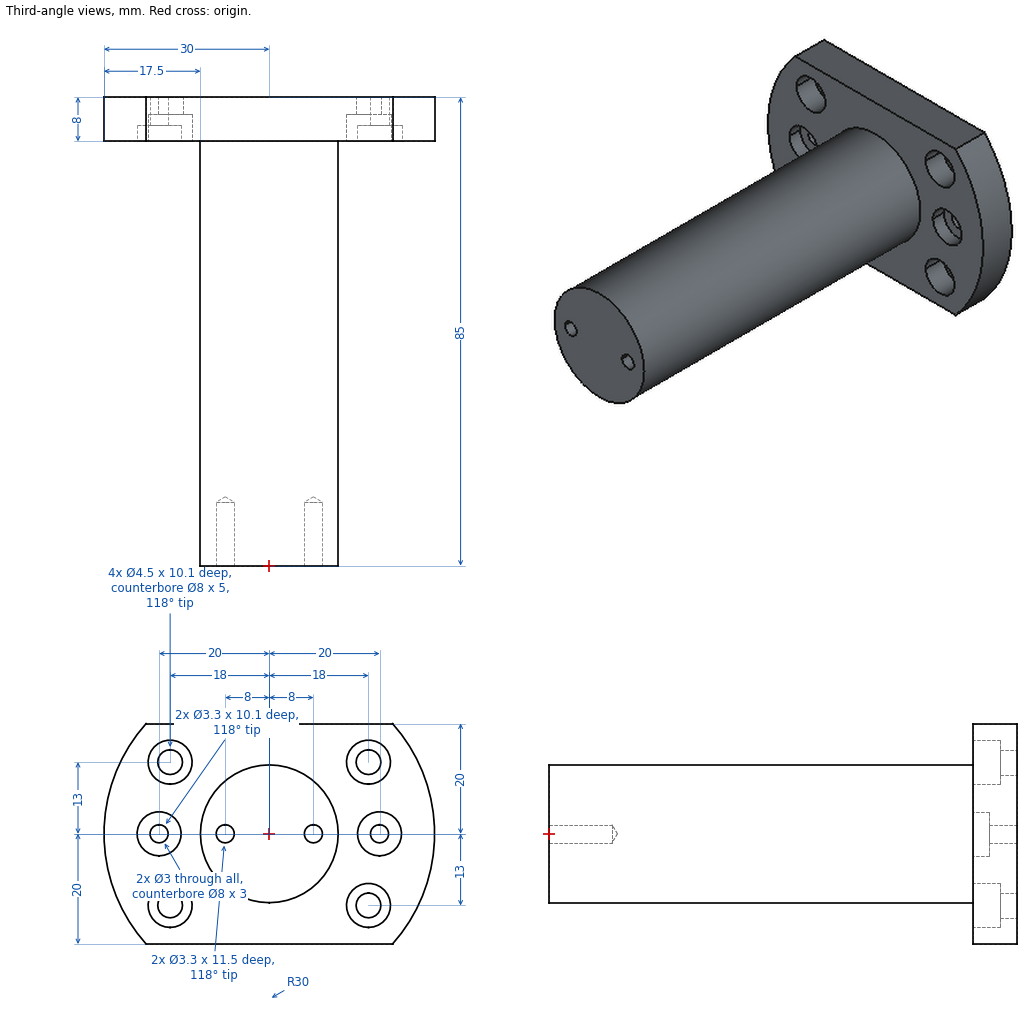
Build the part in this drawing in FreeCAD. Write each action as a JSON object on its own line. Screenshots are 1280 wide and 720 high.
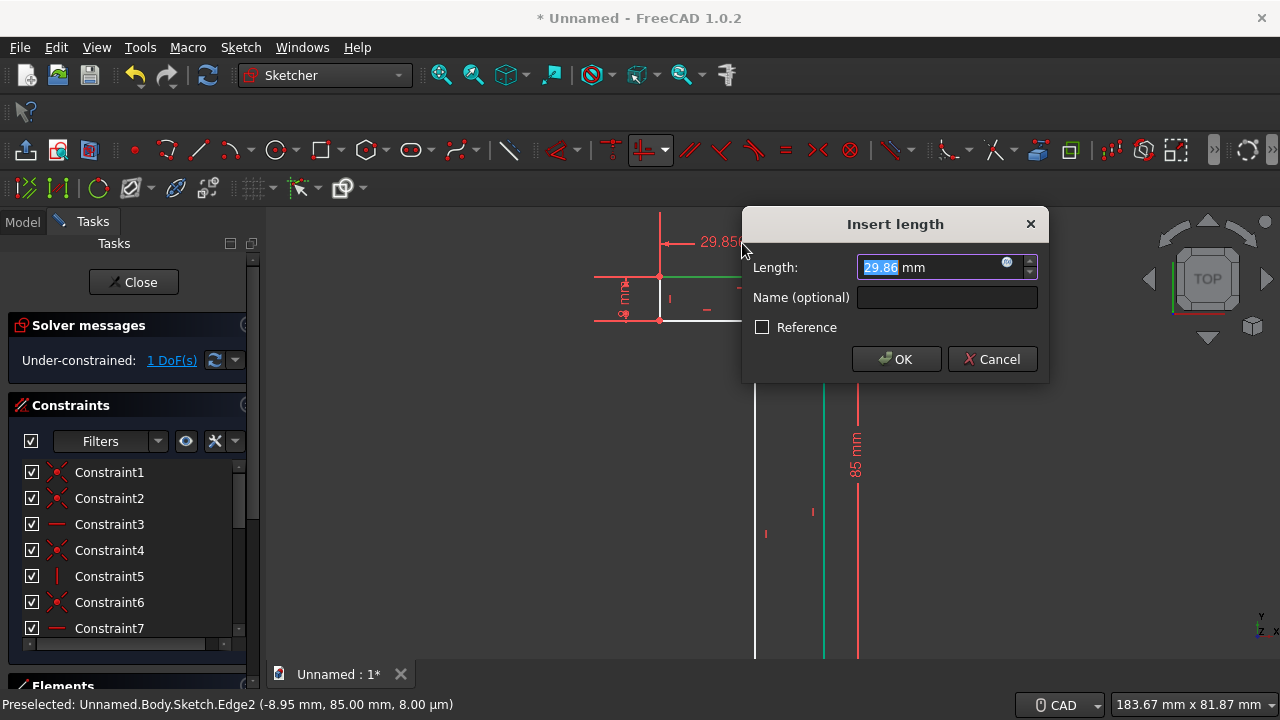
{"action": "type", "text": "30"}
{"action": "key", "text": "Return"}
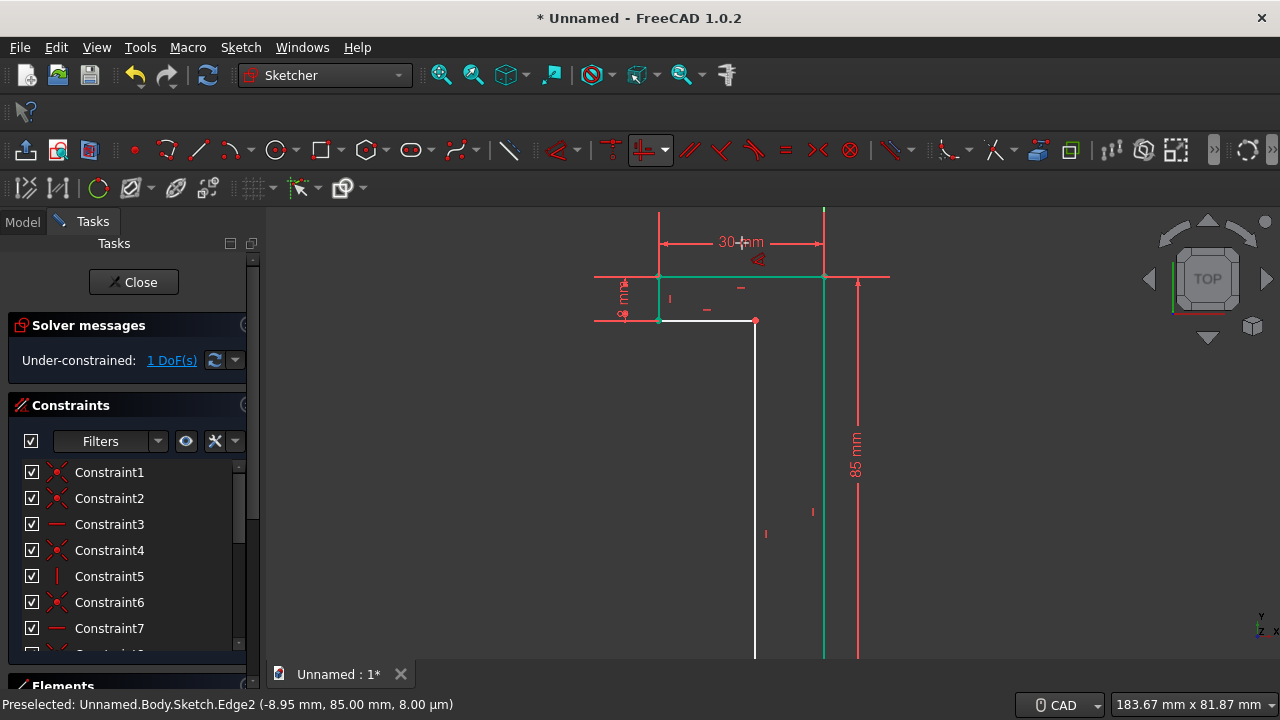
{"action": "left_click", "coordinate": [688, 321]}
{"action": "left_click", "coordinate": [707, 355]}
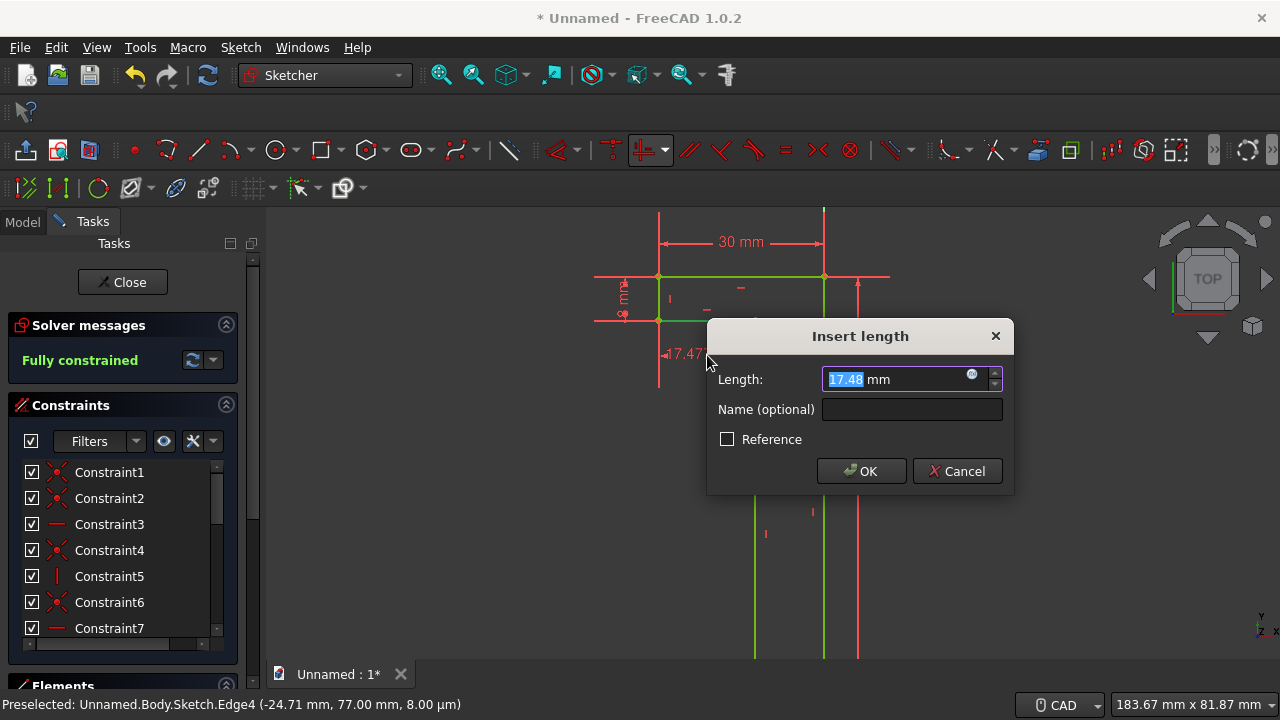
{"action": "type", "text": "17.5"}
{"action": "key", "text": "Return"}
{"action": "key", "text": "Escape"}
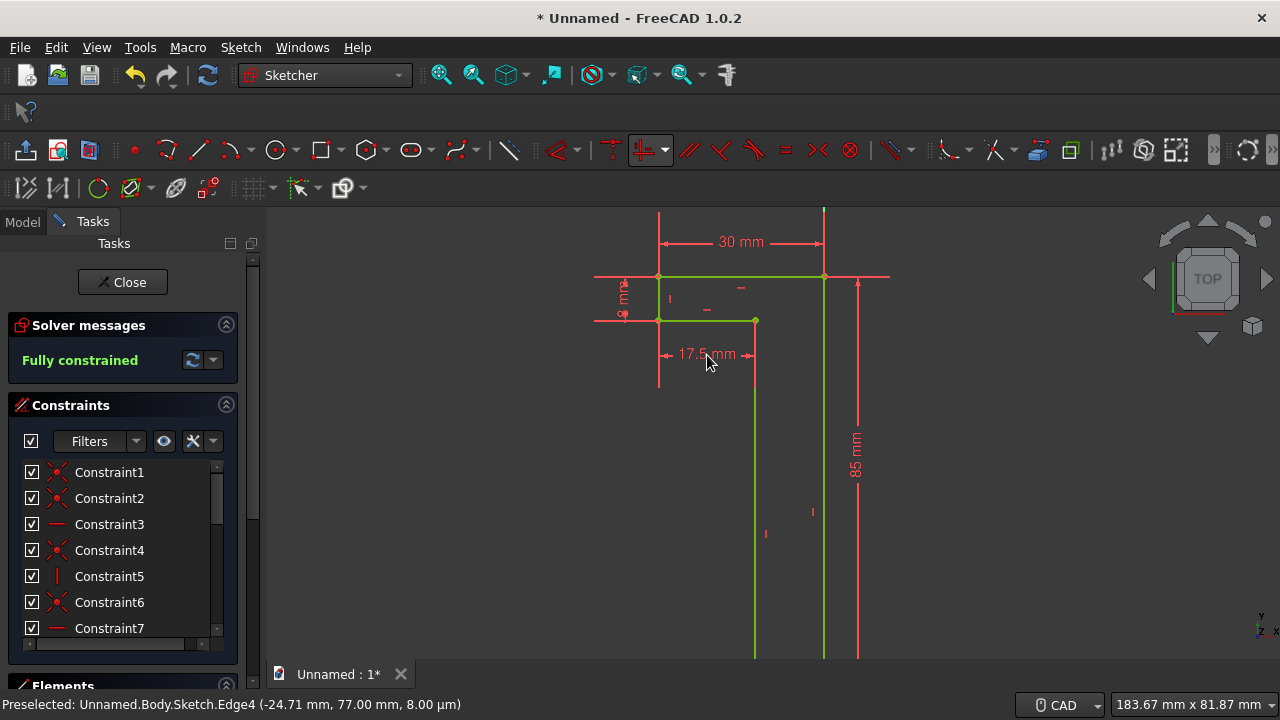
{"action": "left_click", "coordinate": [123, 282]}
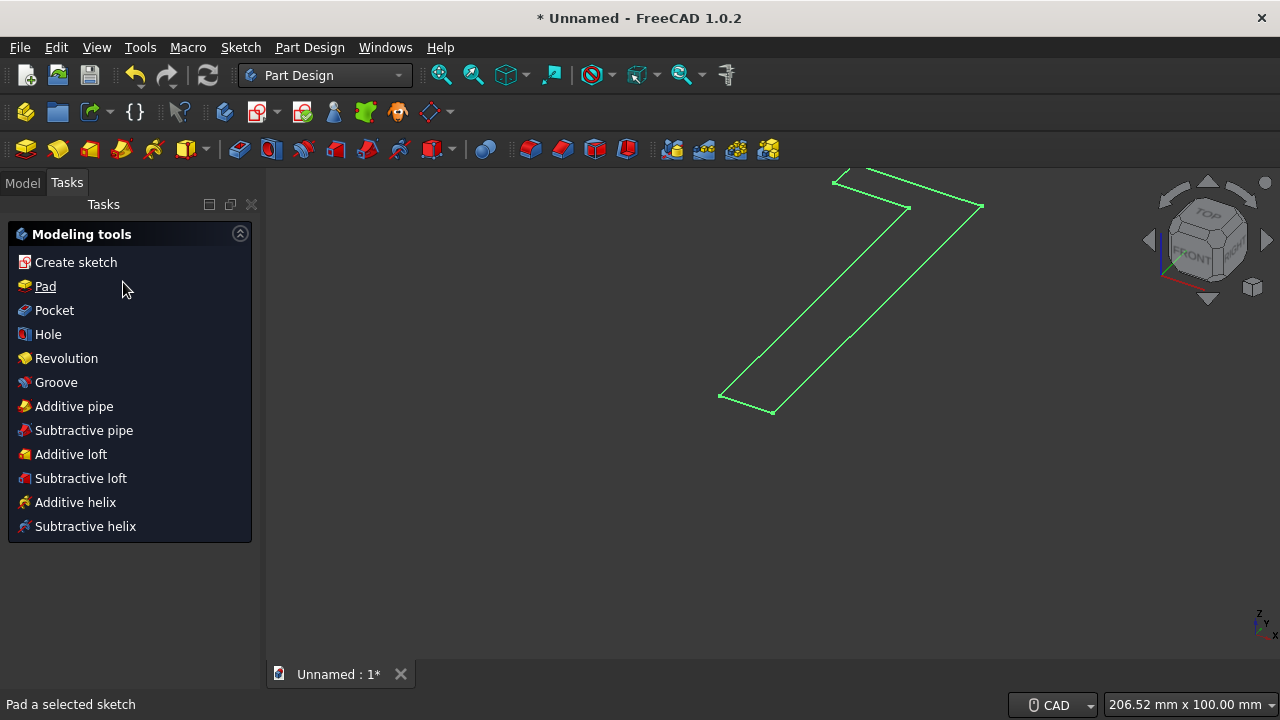
{"action": "left_click", "coordinate": [58, 150]}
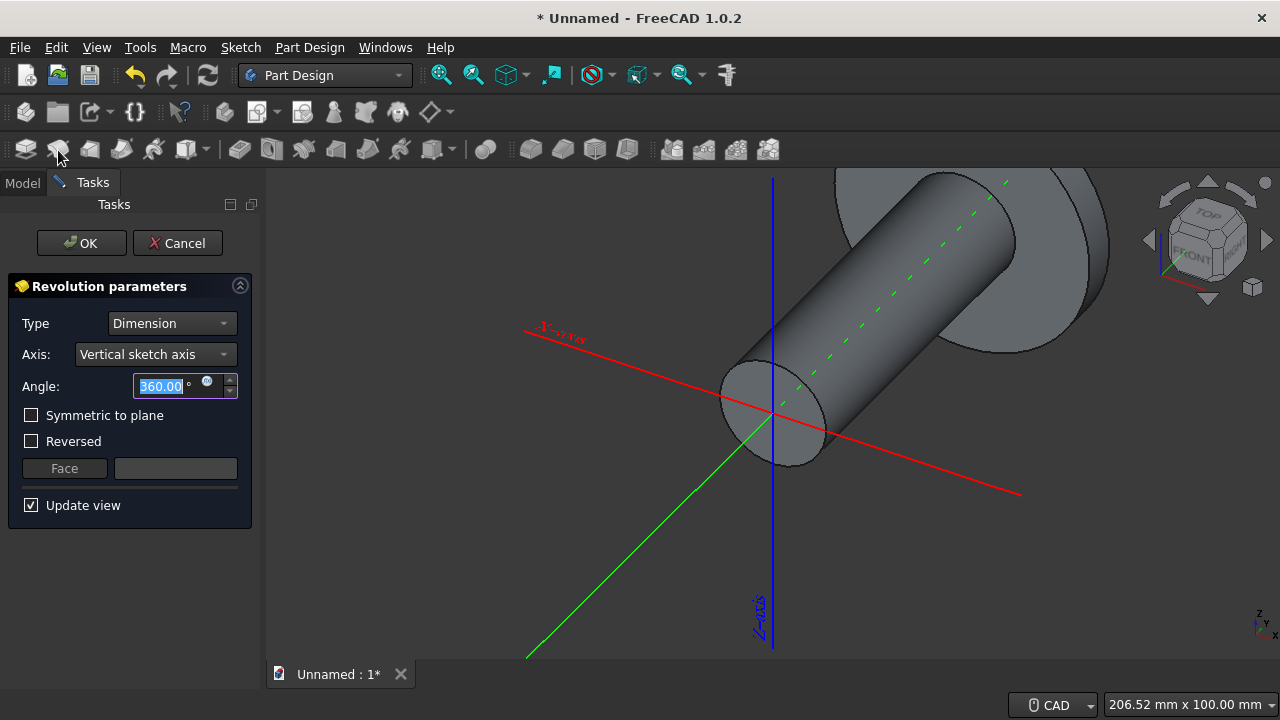
{"action": "left_click", "coordinate": [82, 243]}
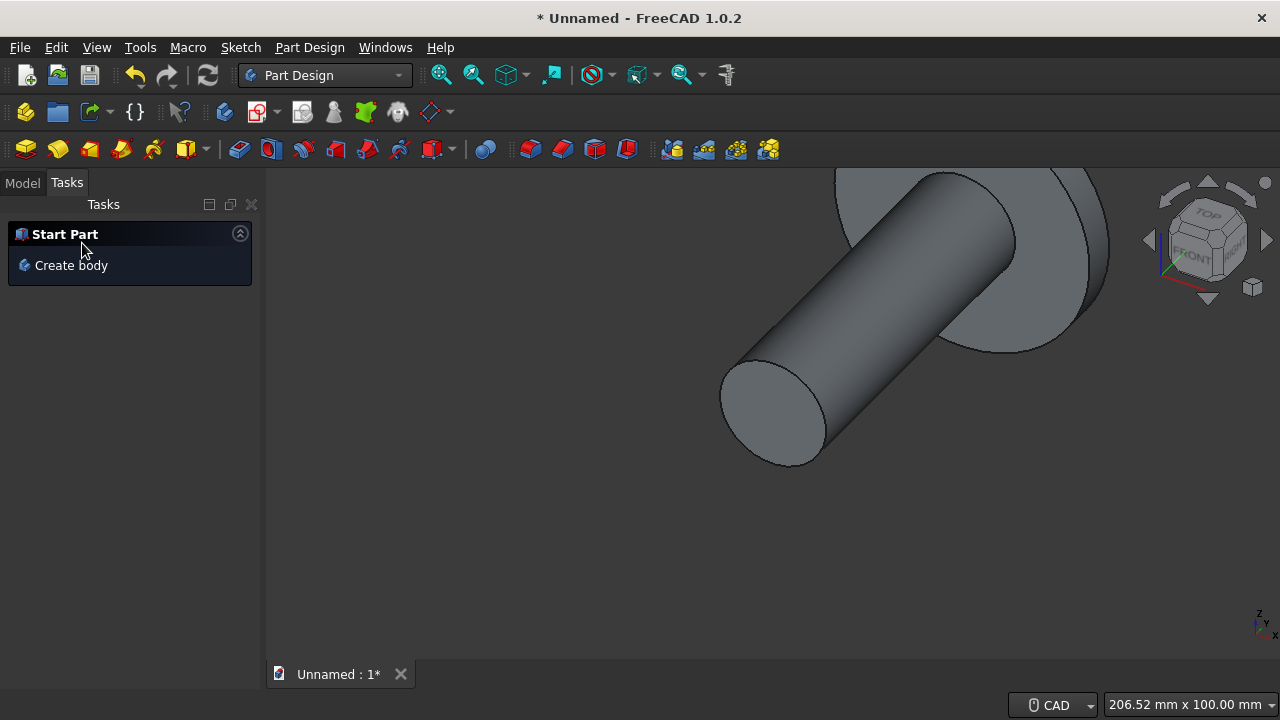
{"action": "left_click", "coordinate": [442, 76]}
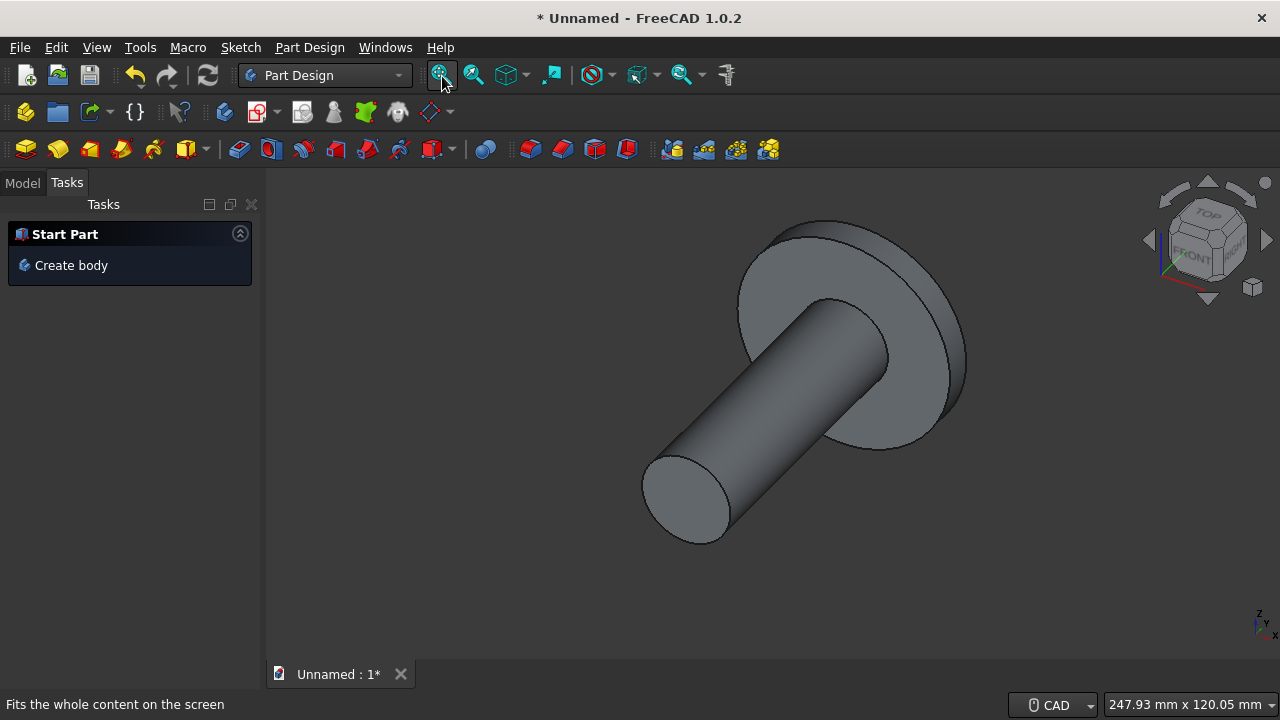
{"action": "left_click", "coordinate": [686, 499]}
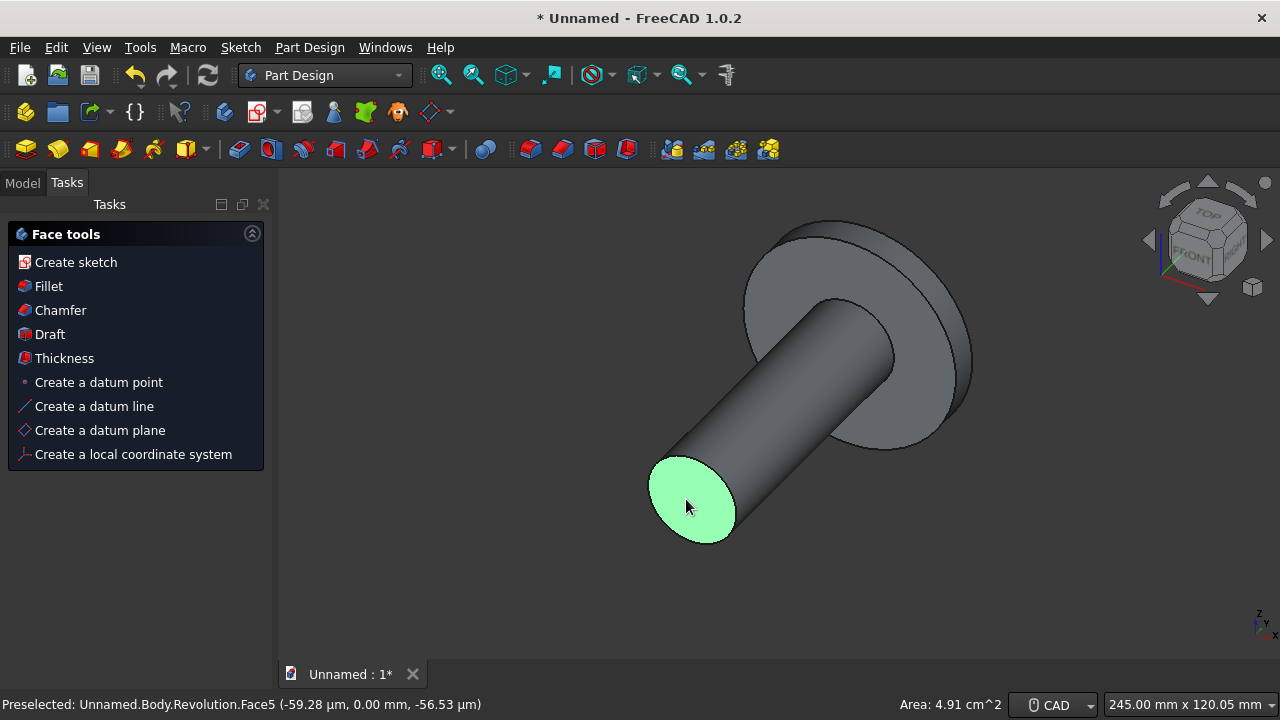
{"action": "left_click", "coordinate": [258, 112]}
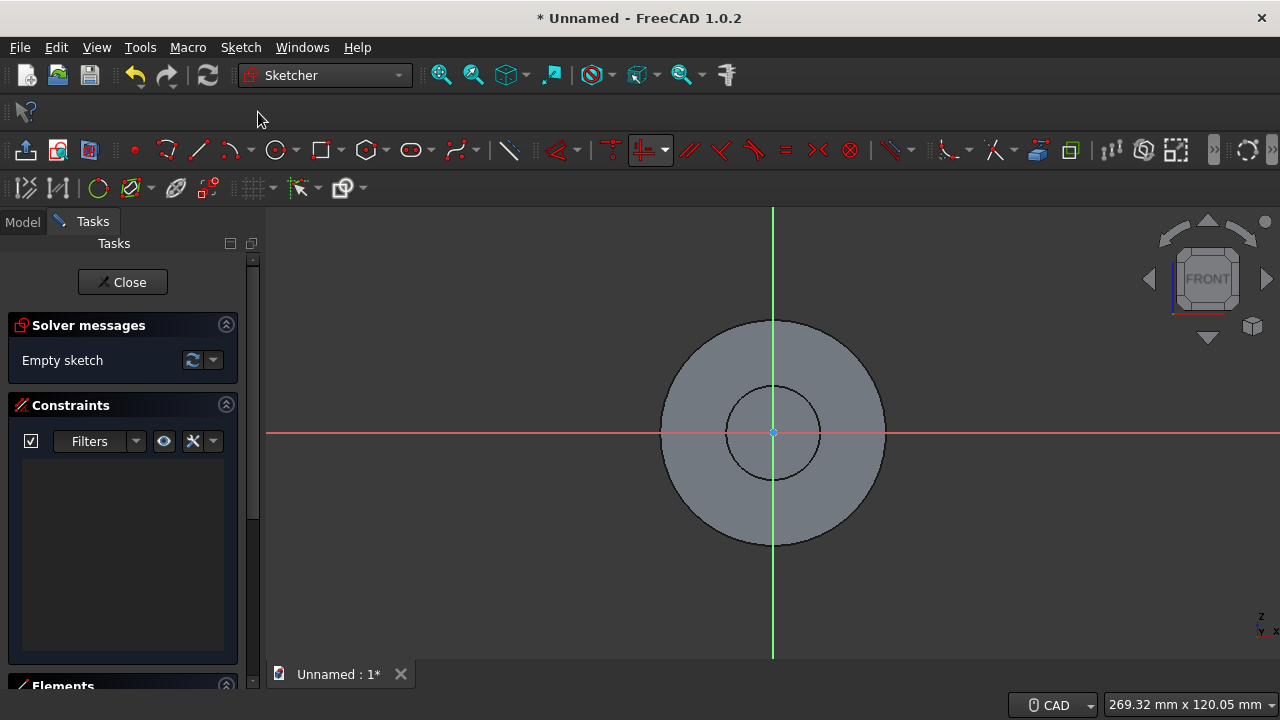
{"action": "scroll", "coordinate": [784, 433], "scroll_direction": "up", "scroll_amount": 10}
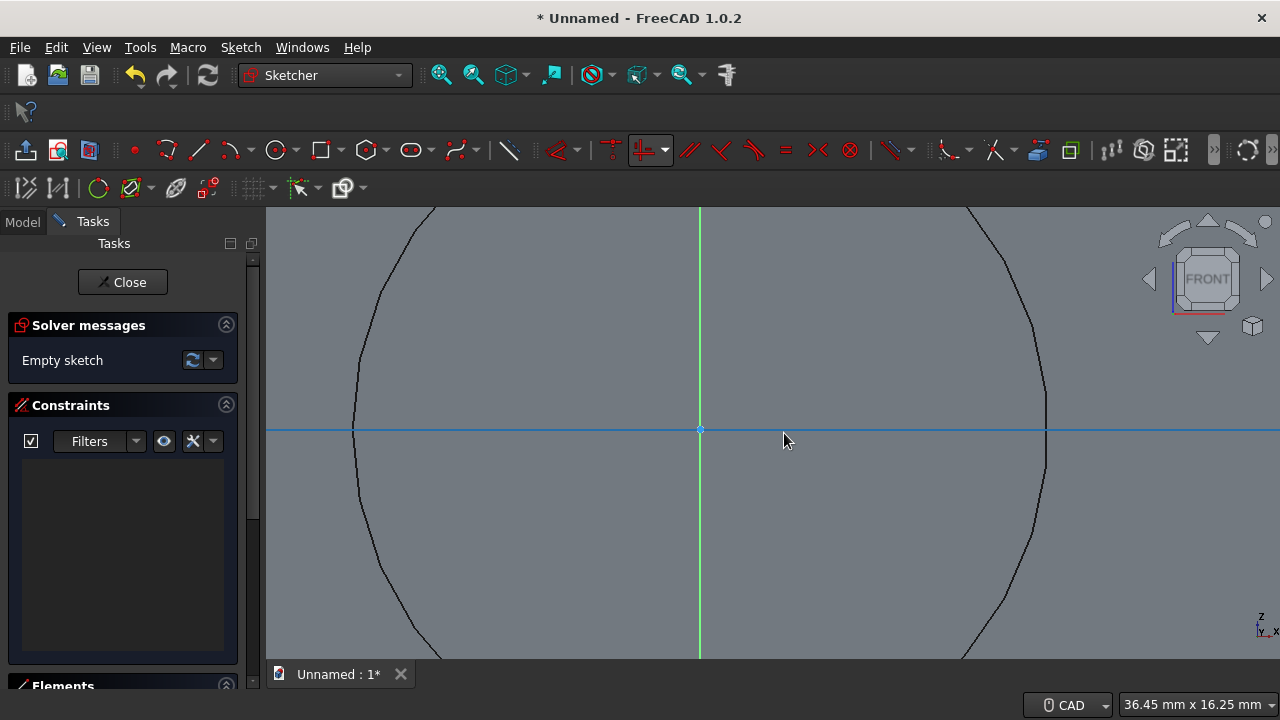
{"action": "left_click", "coordinate": [276, 150]}